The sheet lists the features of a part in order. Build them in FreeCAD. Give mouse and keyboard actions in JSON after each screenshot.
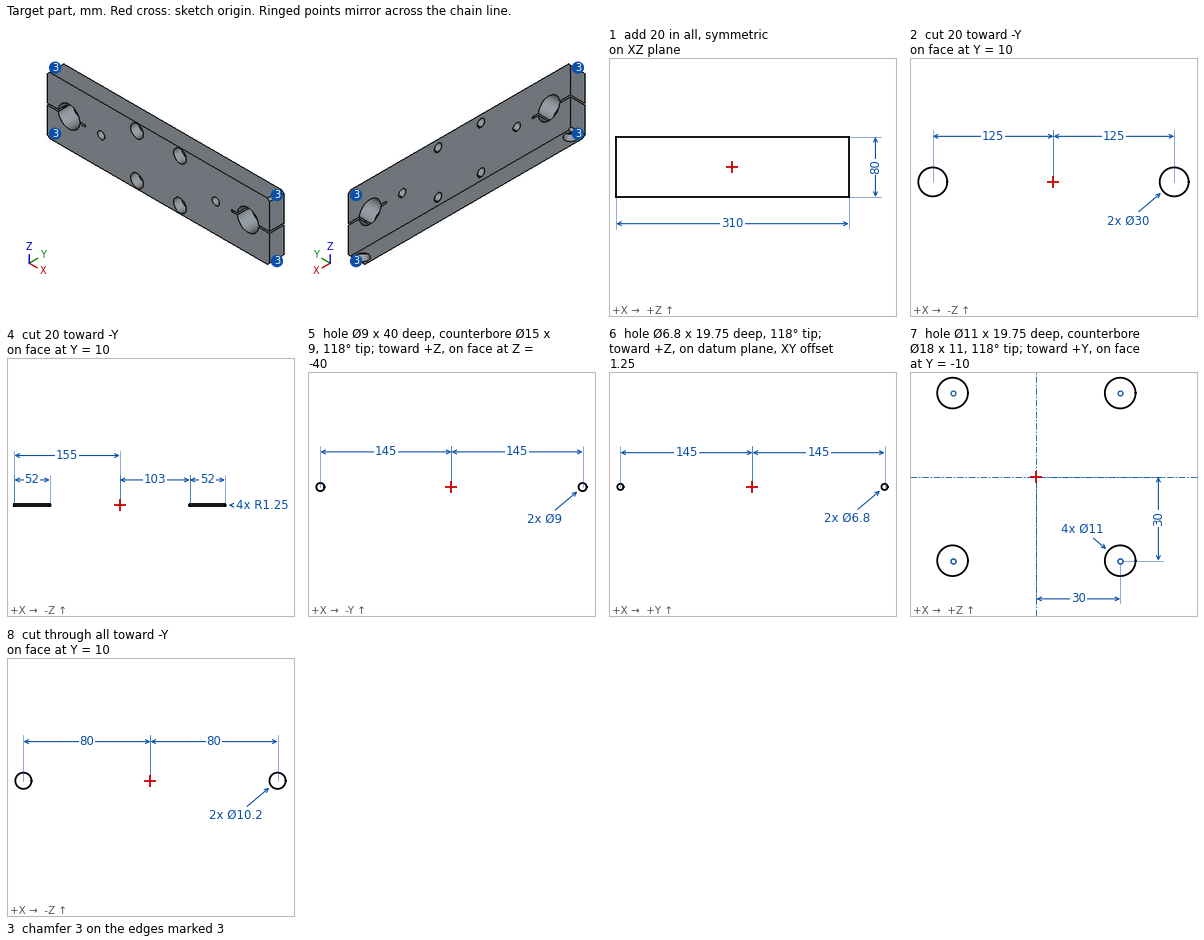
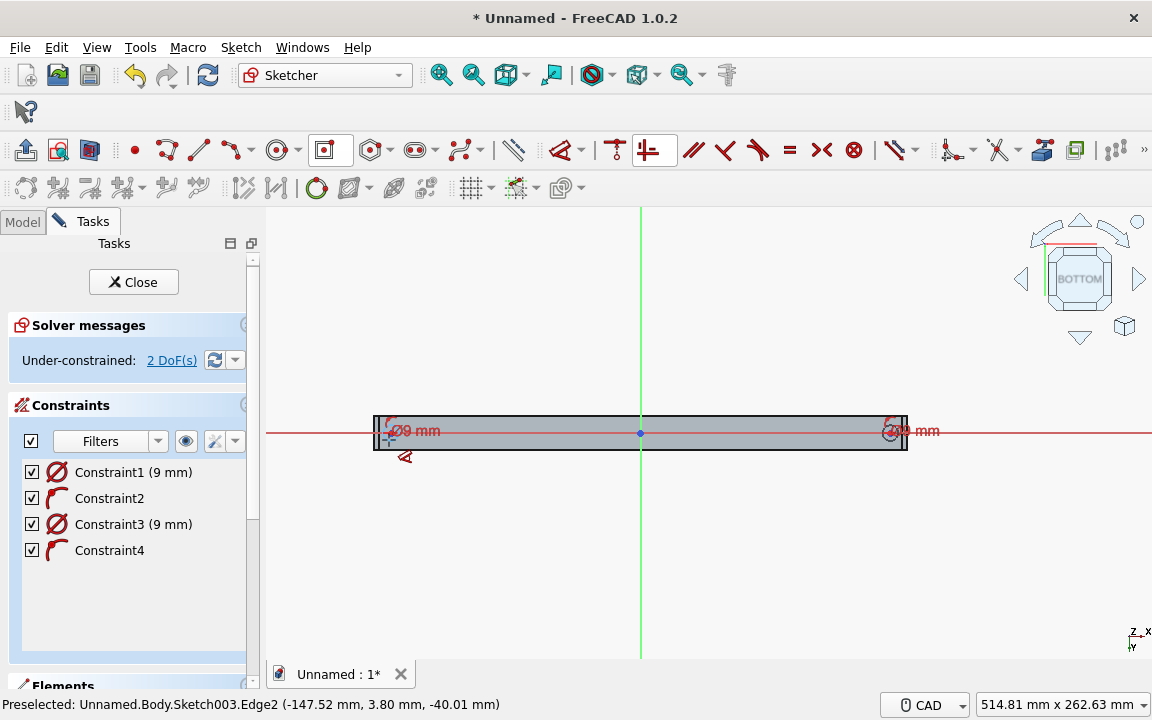
{"action": "left_click", "coordinate": [890, 433]}
{"action": "left_click", "coordinate": [766, 467]}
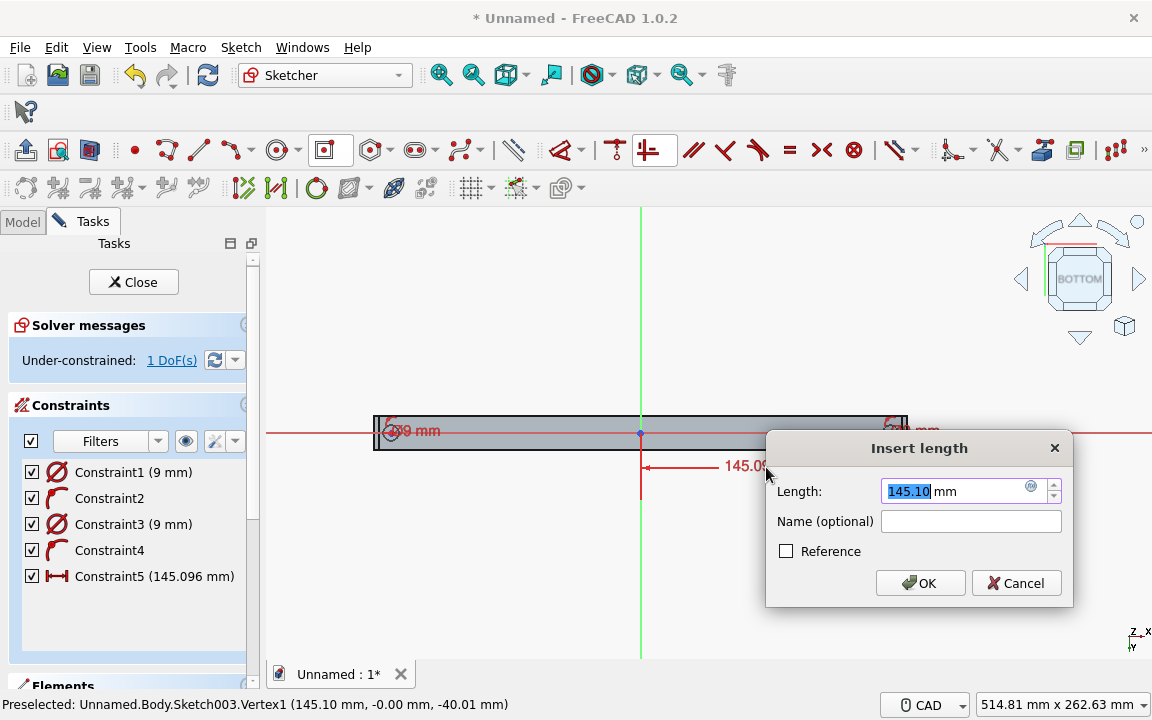
{"action": "type", "text": "145"}
{"action": "key", "text": "Return"}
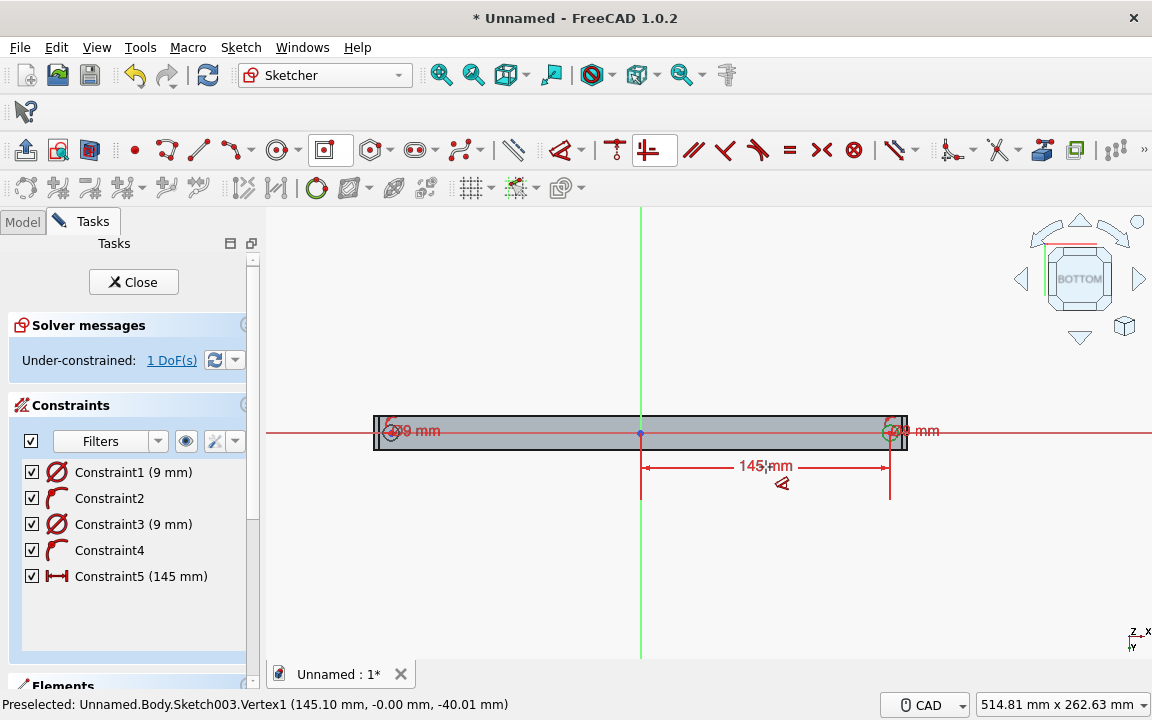
{"action": "left_click", "coordinate": [391, 433]}
{"action": "left_click", "coordinate": [516, 467]}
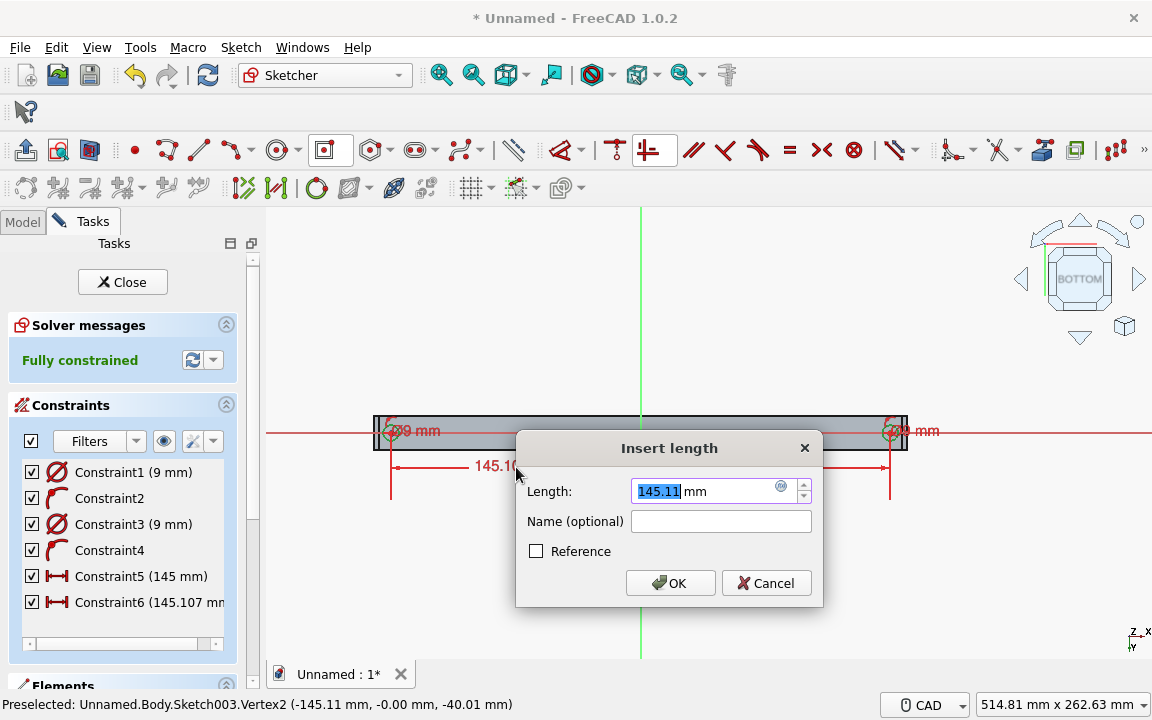
{"action": "type", "text": "145"}
{"action": "key", "text": "Return"}
{"action": "key", "text": "Escape"}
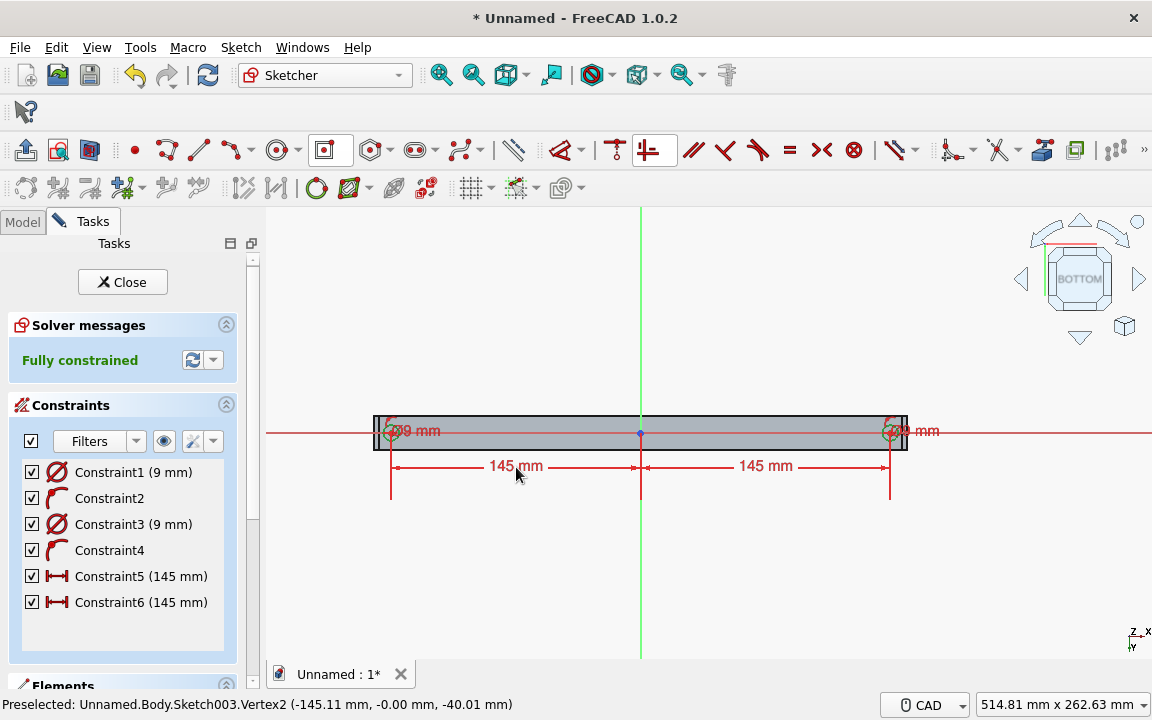
{"action": "left_click", "coordinate": [123, 282]}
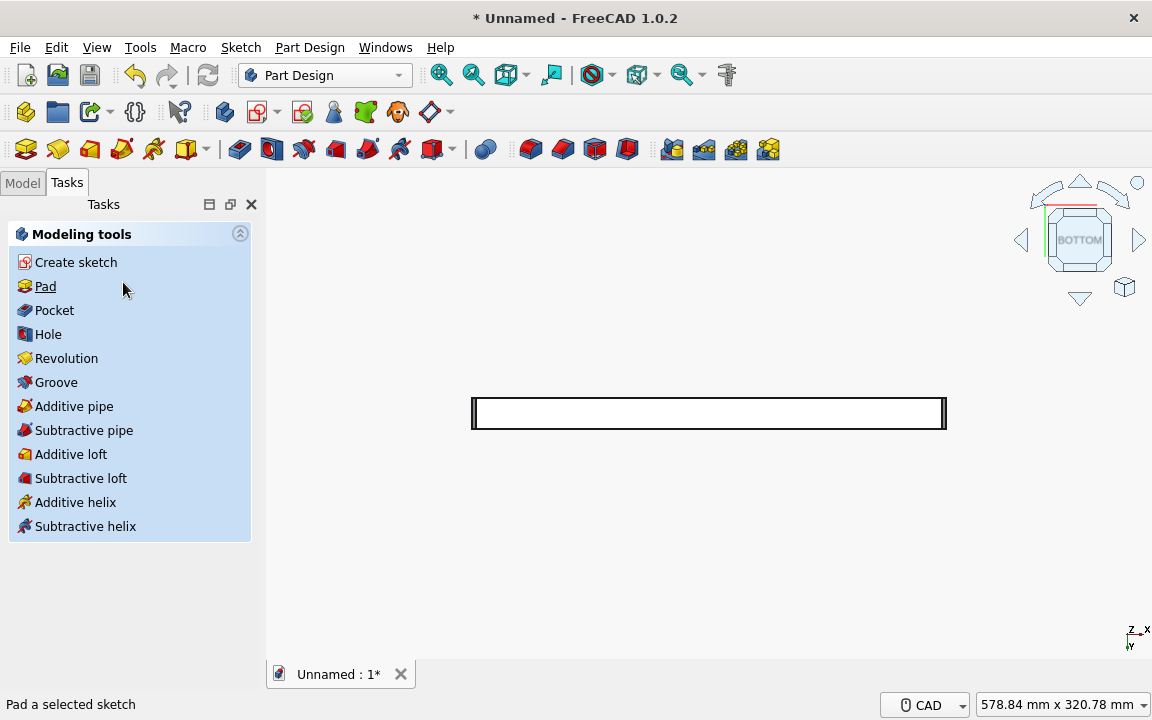
{"action": "left_click", "coordinate": [272, 150]}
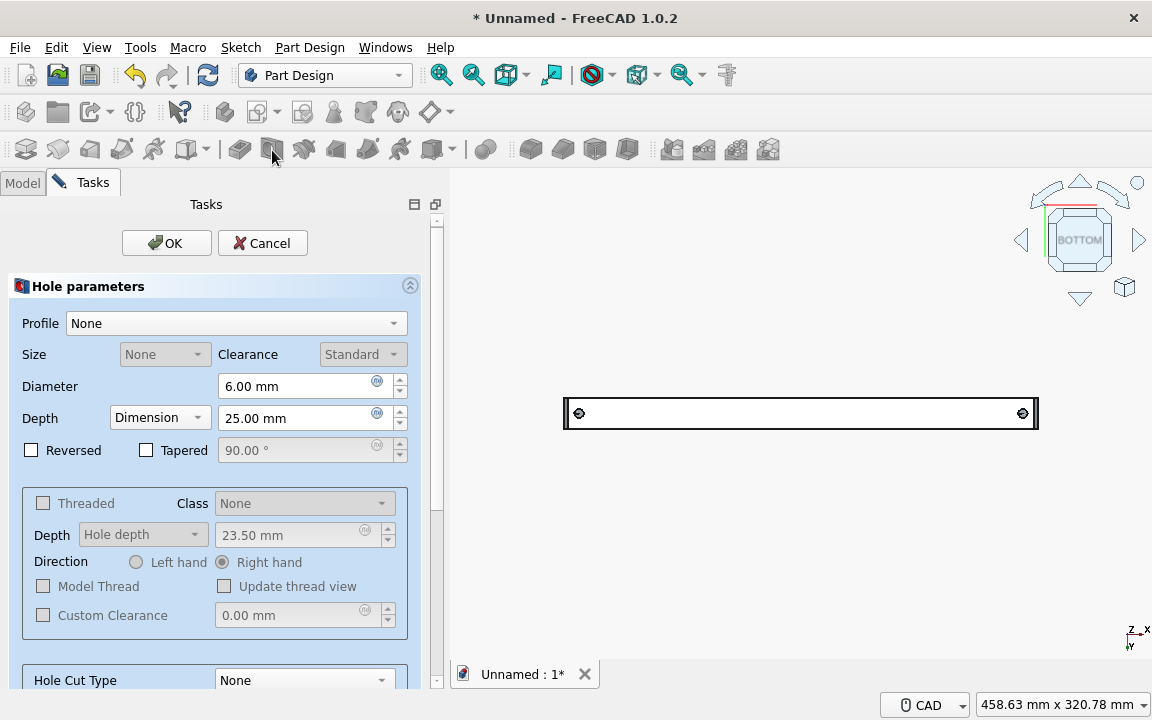
{"action": "triple_click", "coordinate": [305, 386]}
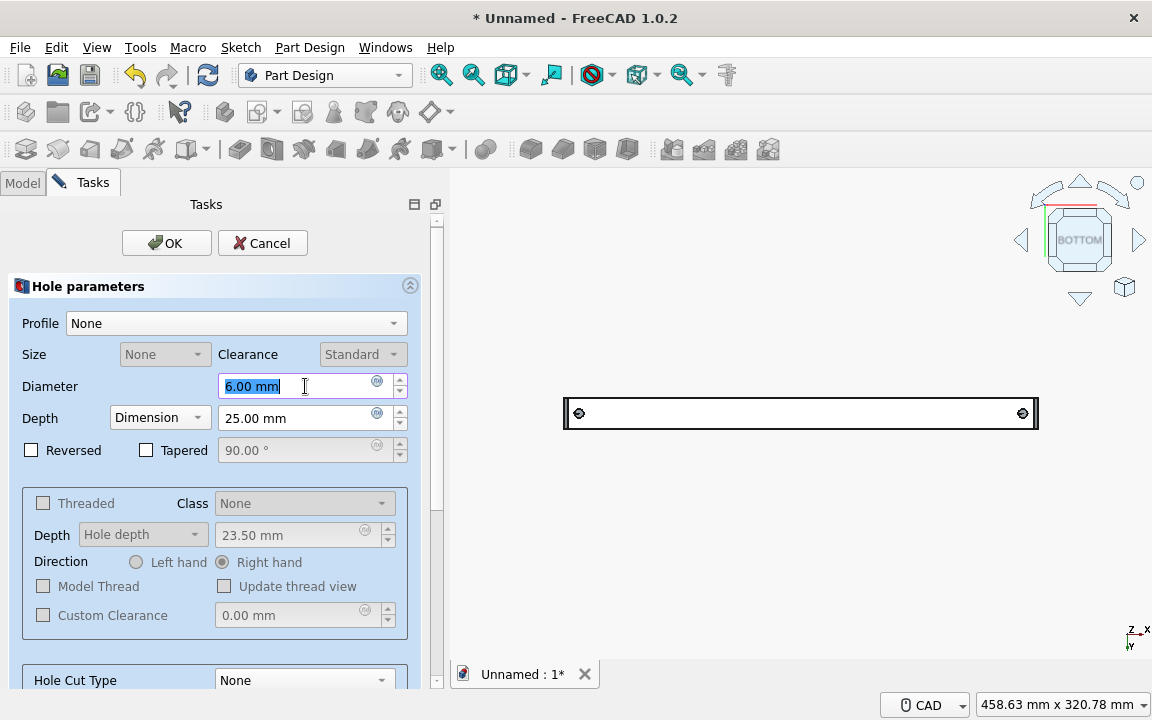
{"action": "type", "text": "9"}
{"action": "key", "text": "Tab"}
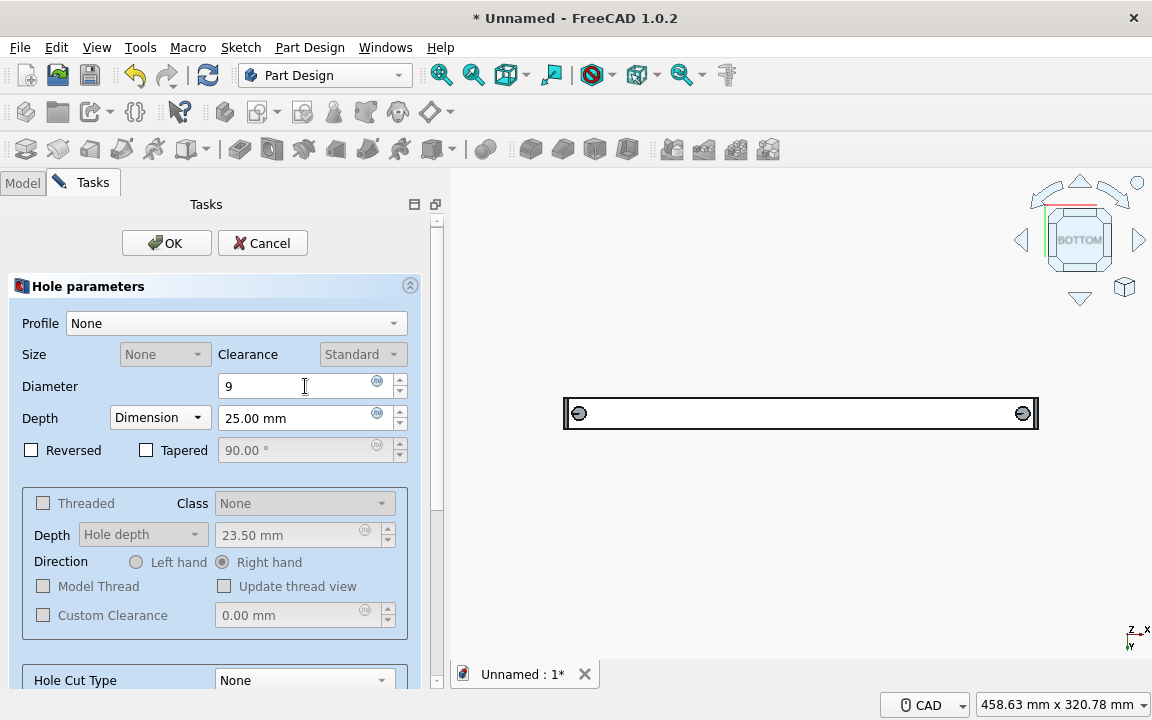
{"action": "triple_click", "coordinate": [305, 418]}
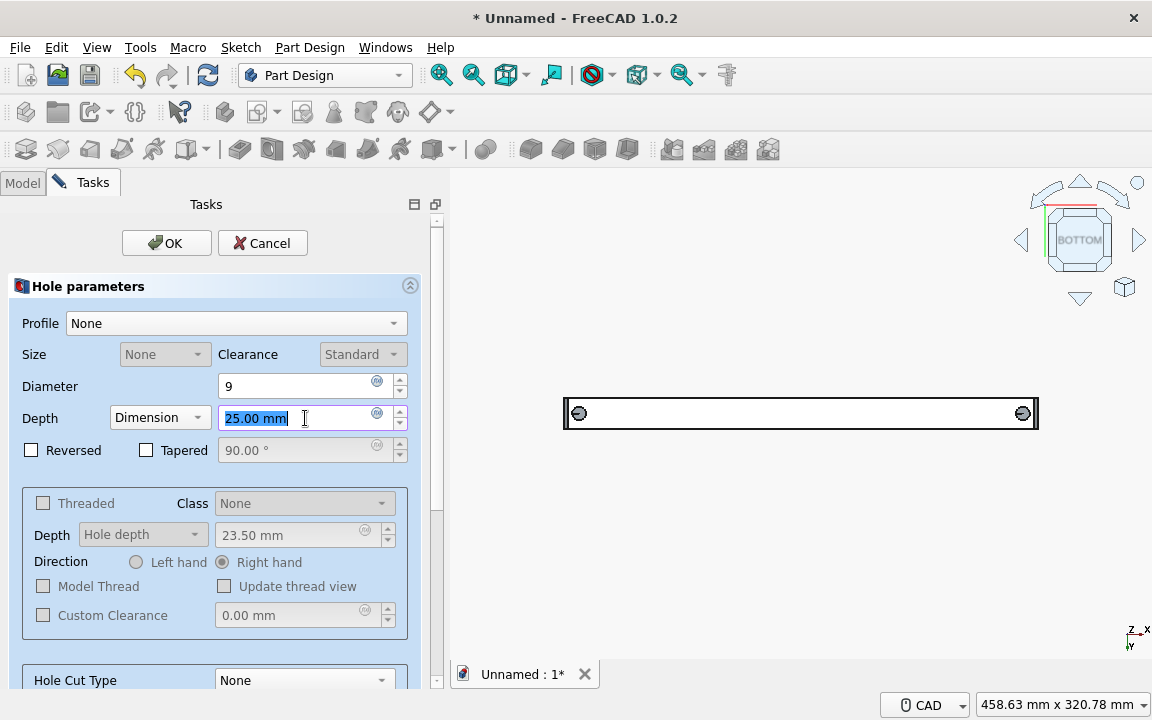
{"action": "type", "text": "40"}
{"action": "key", "text": "Tab"}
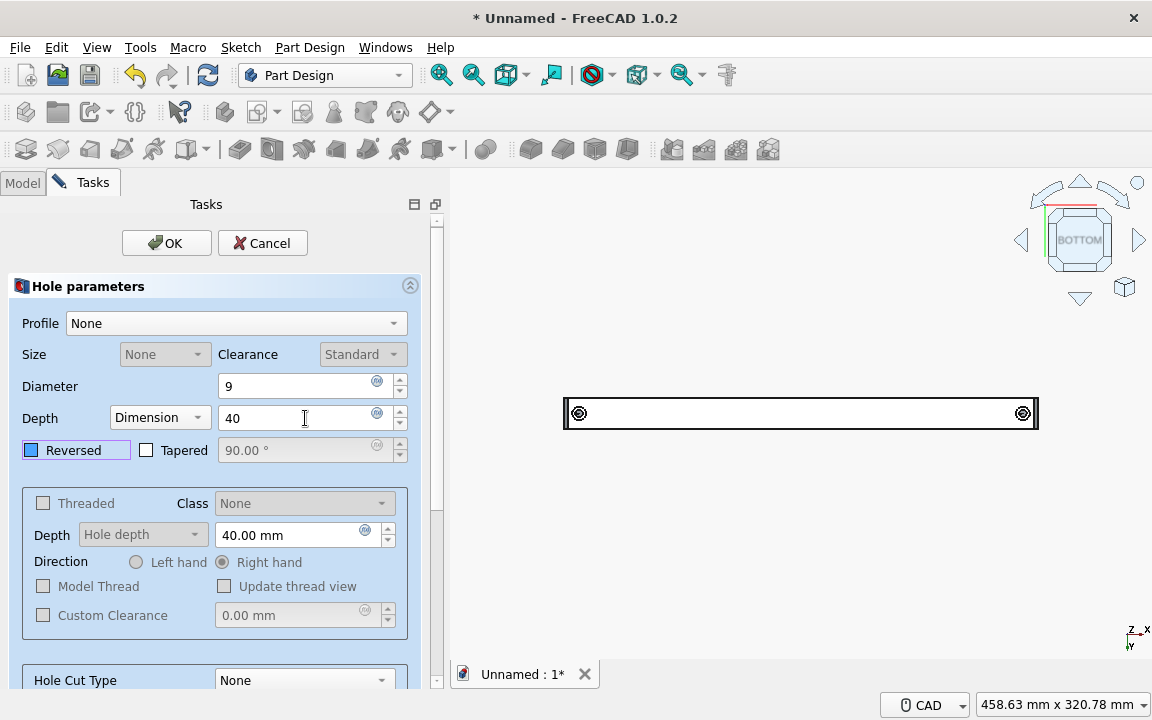
{"action": "scroll", "coordinate": [437, 451], "scroll_direction": "down", "scroll_amount": 2}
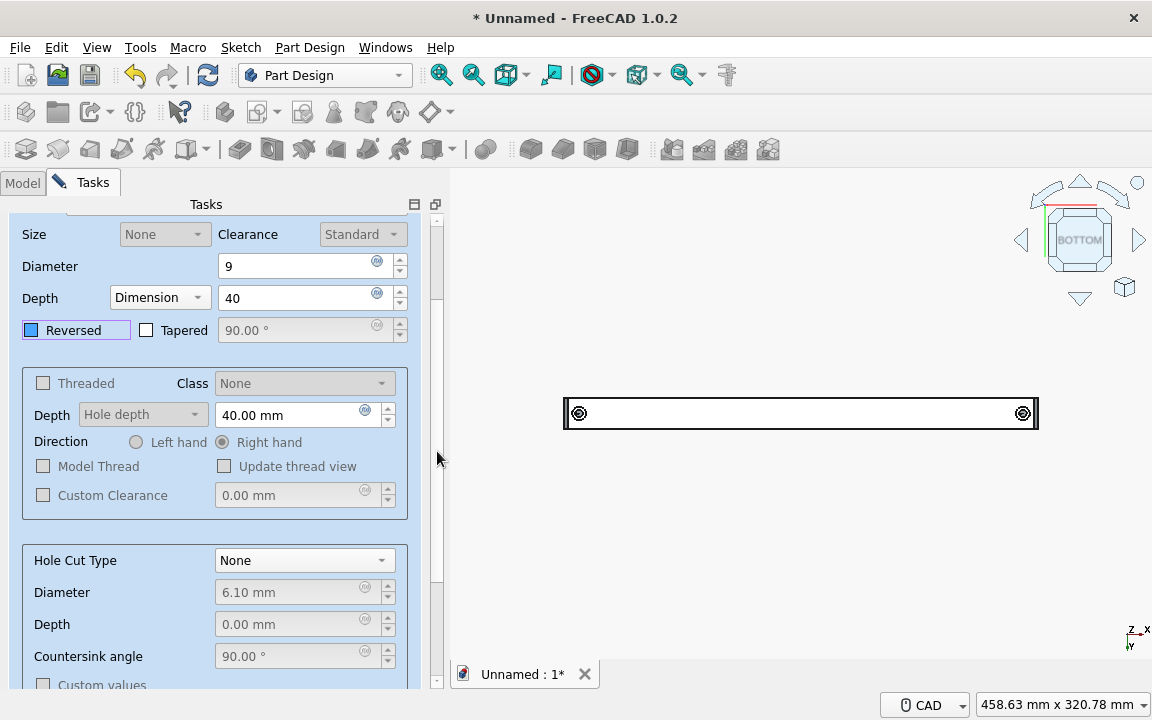
{"action": "left_click", "coordinate": [306, 560]}